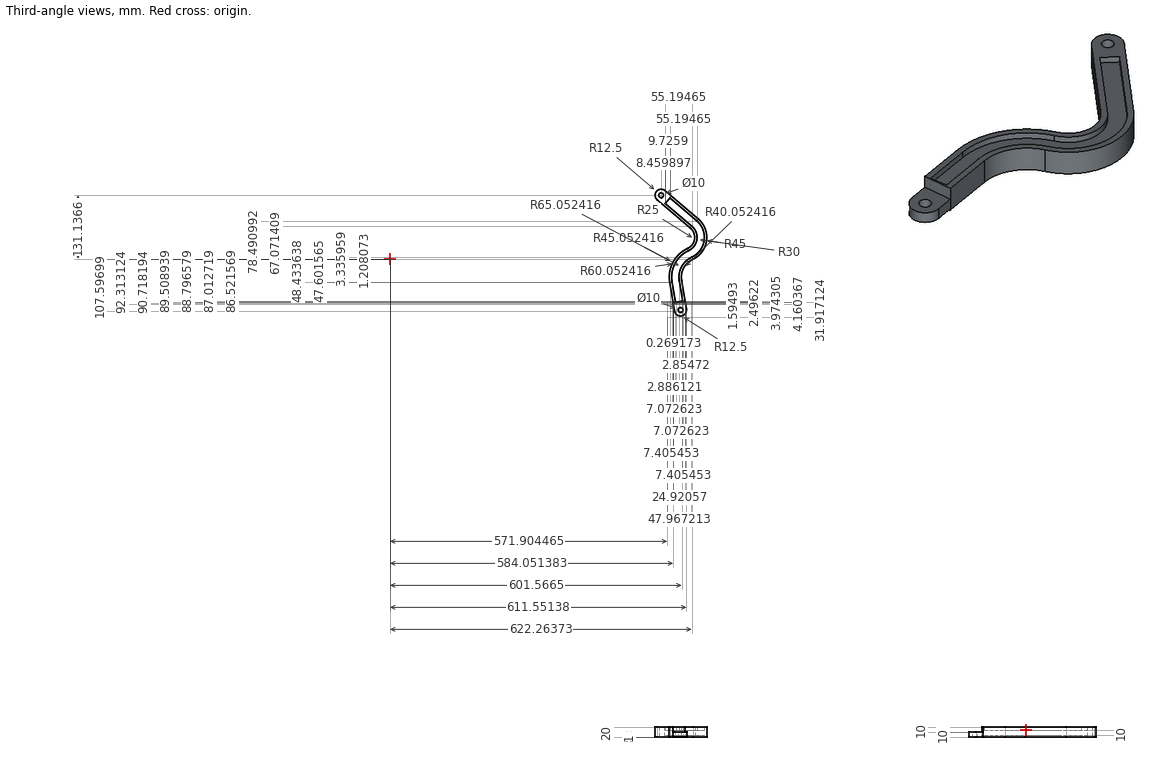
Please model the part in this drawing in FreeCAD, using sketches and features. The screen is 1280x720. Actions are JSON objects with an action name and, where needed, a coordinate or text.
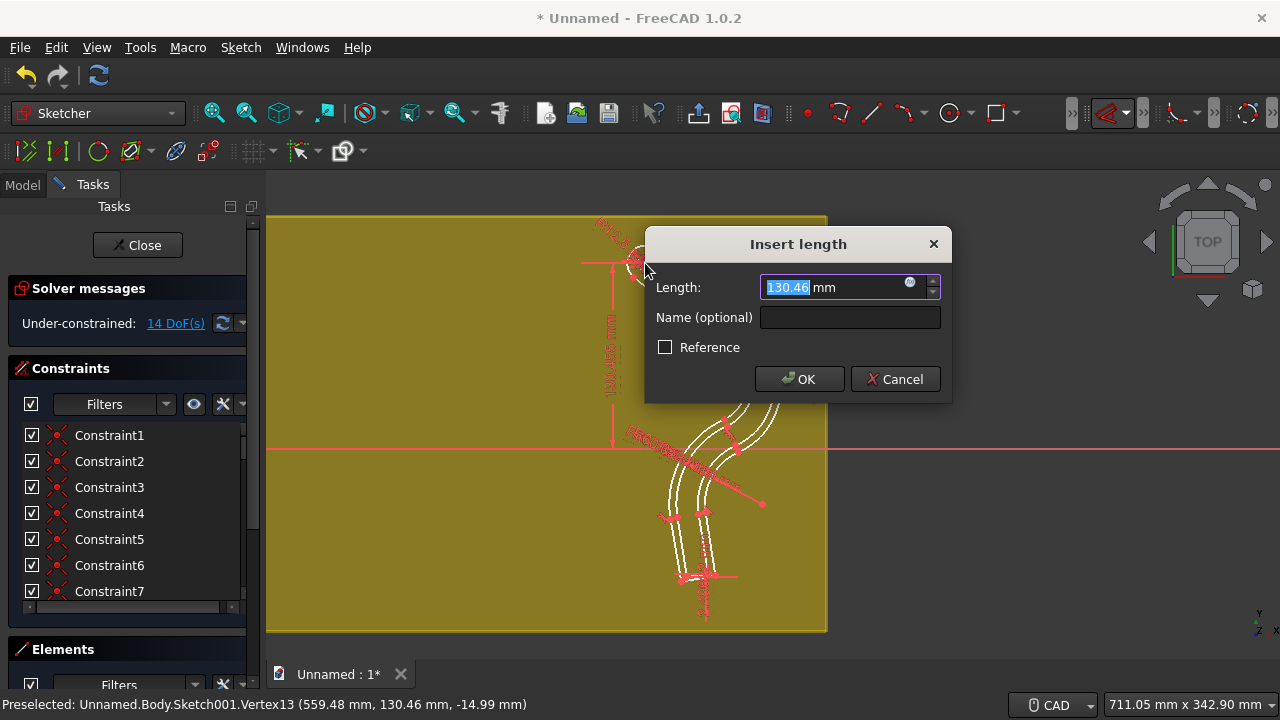
{"action": "type", "text": "131.1366"}
{"action": "key", "text": "Return"}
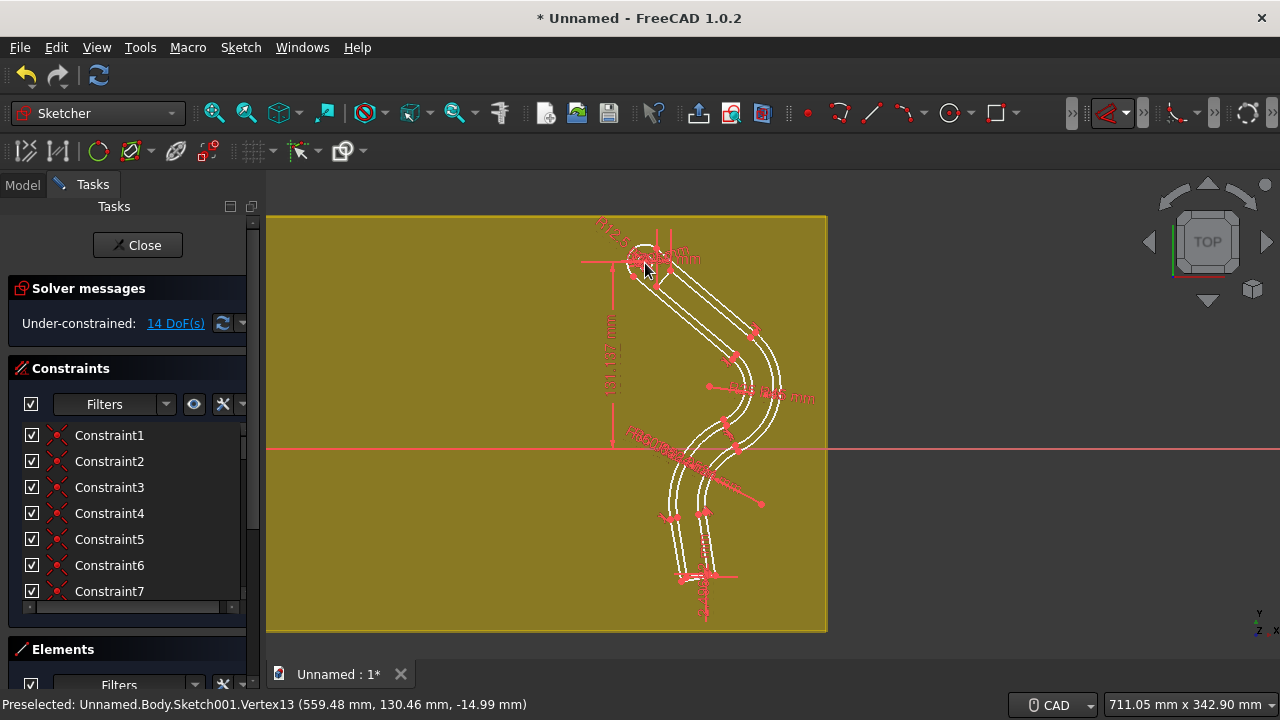
{"action": "scroll", "coordinate": [706, 513], "scroll_direction": "up", "scroll_amount": 3}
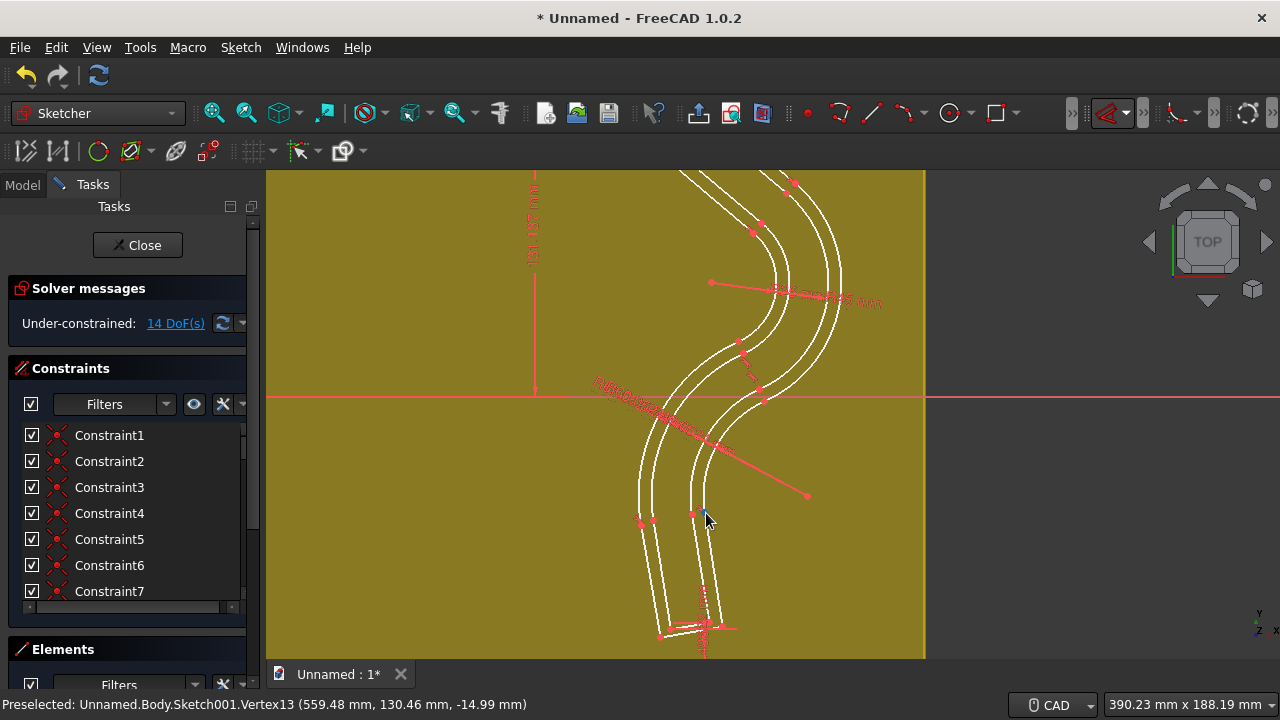
{"action": "left_click", "coordinate": [705, 512]}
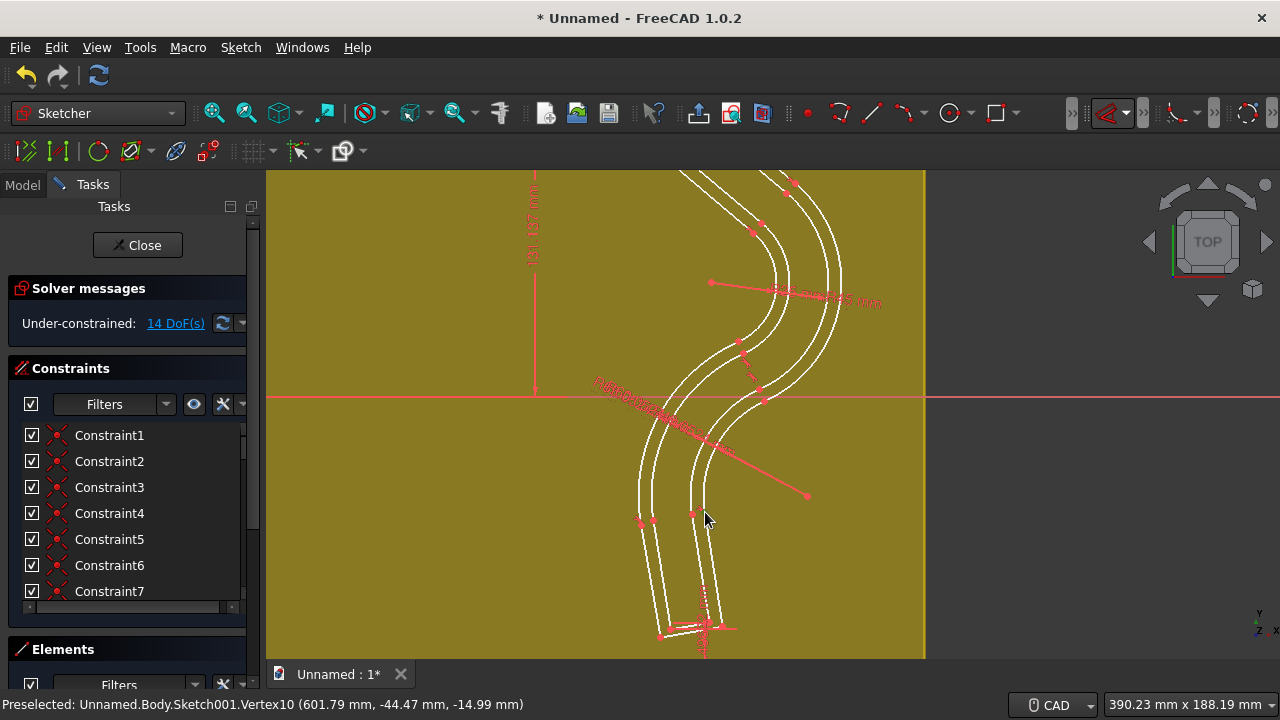
{"action": "left_click", "coordinate": [1128, 114]}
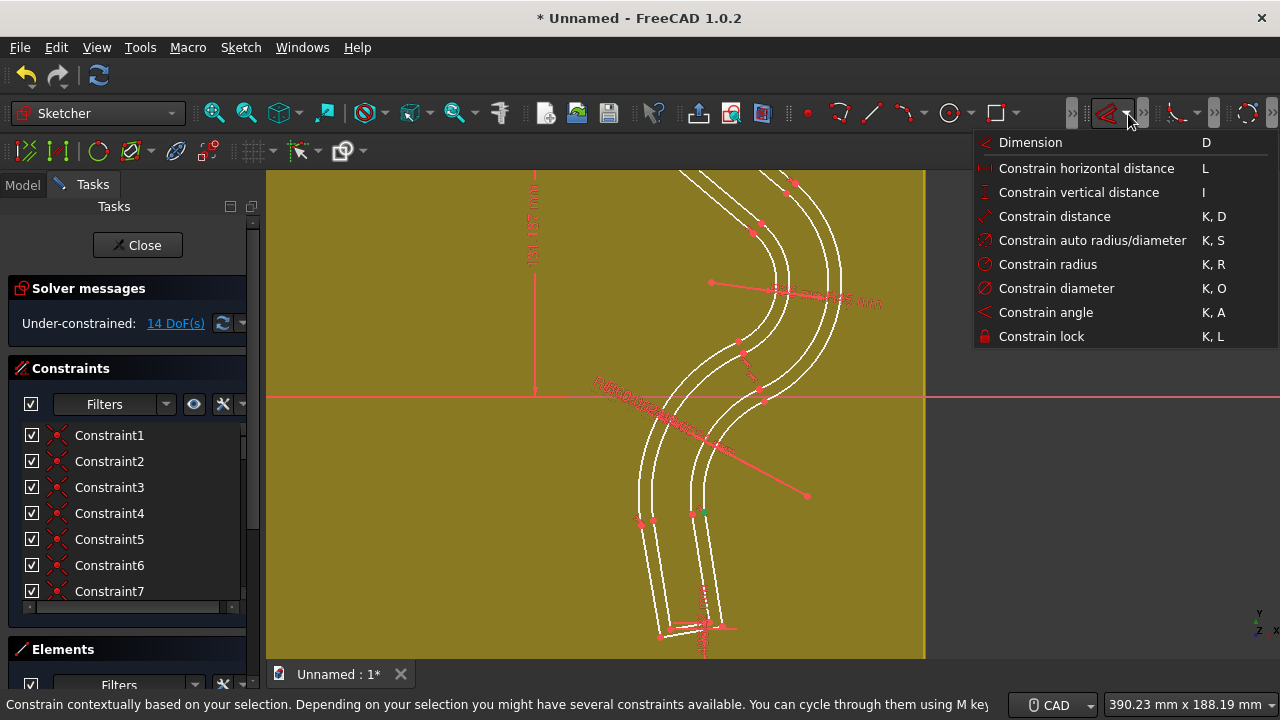
{"action": "left_click", "coordinate": [1126, 168]}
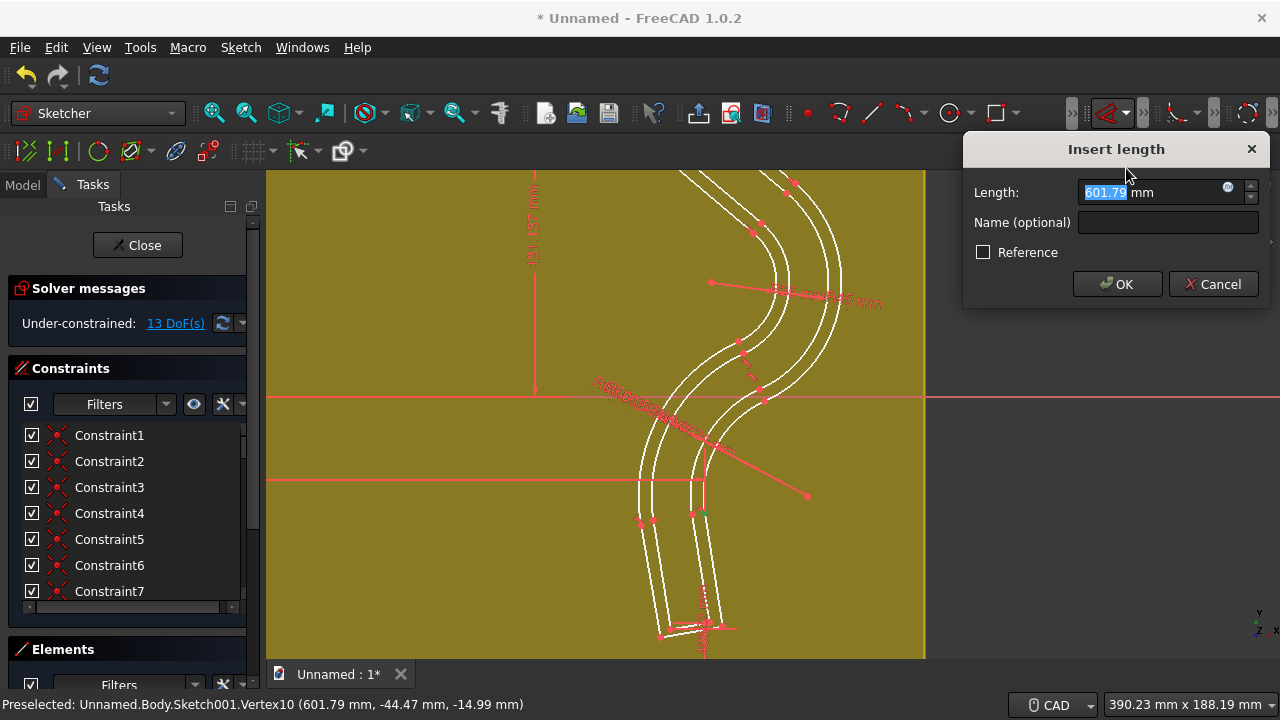
{"action": "type", "text": "601.5665"}
{"action": "key", "text": "Return"}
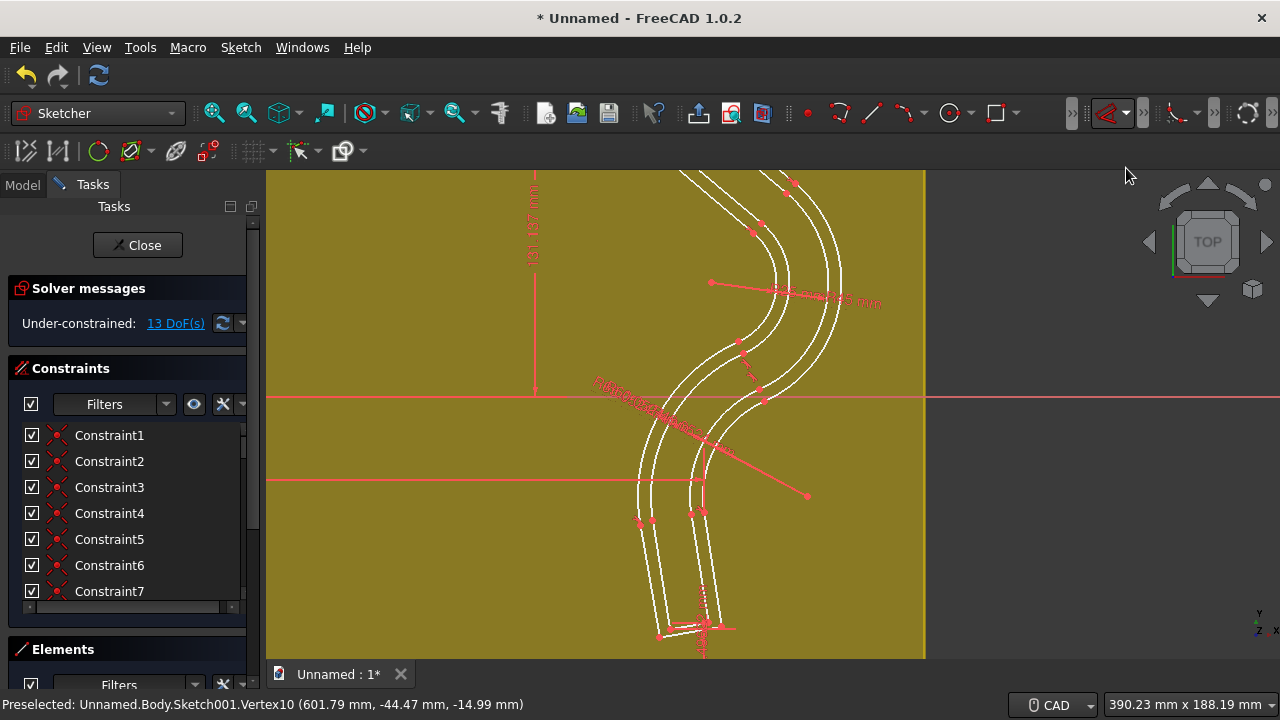
{"action": "scroll", "coordinate": [765, 401], "scroll_direction": "up", "scroll_amount": 13}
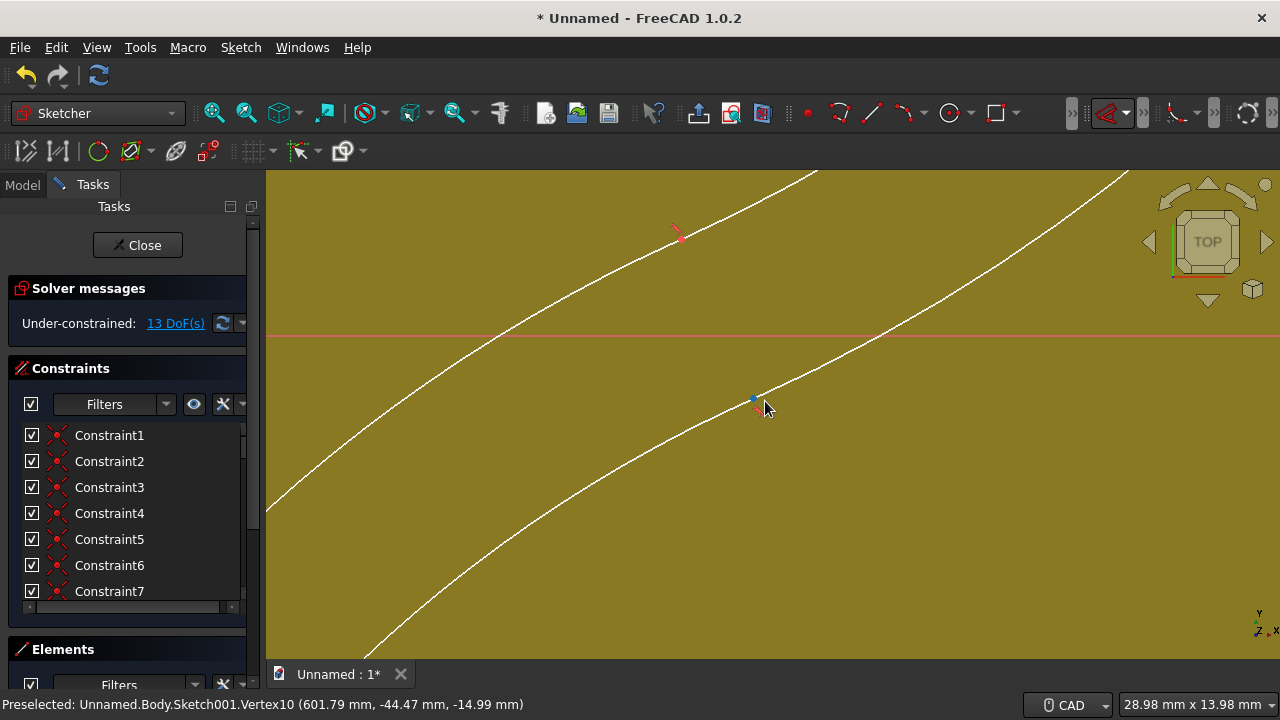
{"action": "left_click", "coordinate": [753, 399]}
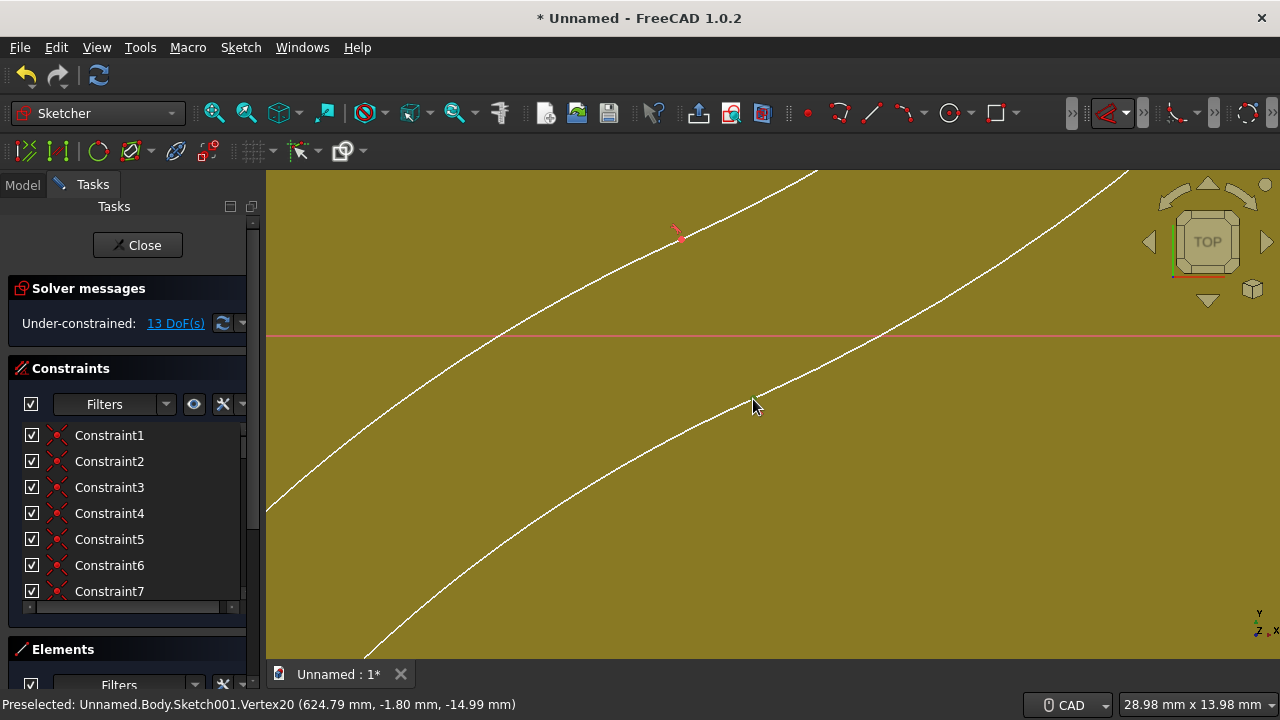
{"action": "left_click", "coordinate": [1128, 114]}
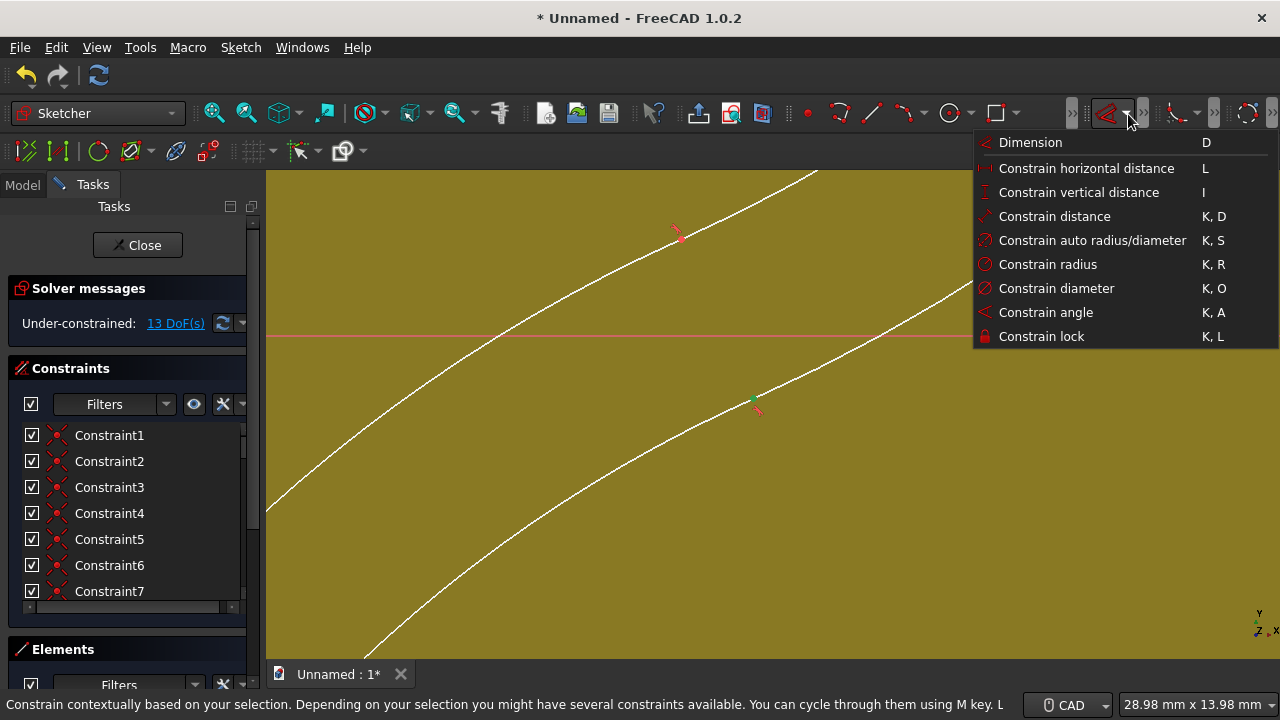
{"action": "left_click", "coordinate": [1126, 192]}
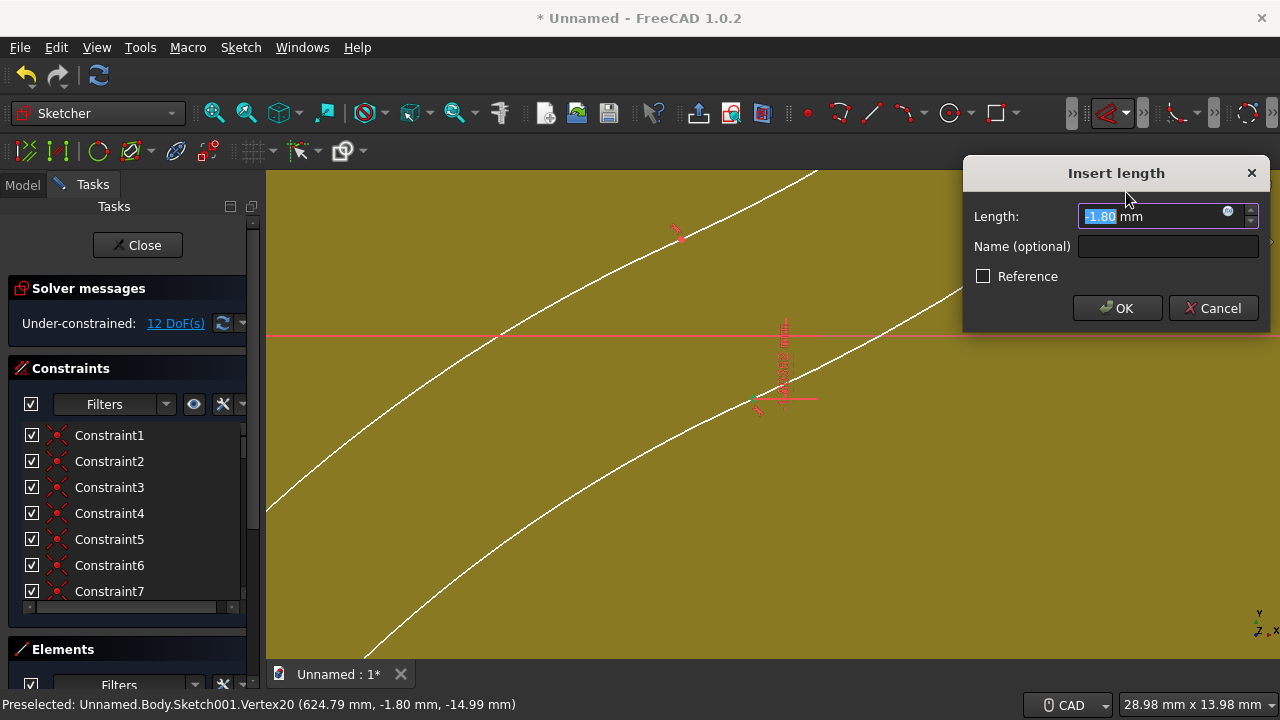
{"action": "type", "text": "-1.208073"}
{"action": "key", "text": "Return"}